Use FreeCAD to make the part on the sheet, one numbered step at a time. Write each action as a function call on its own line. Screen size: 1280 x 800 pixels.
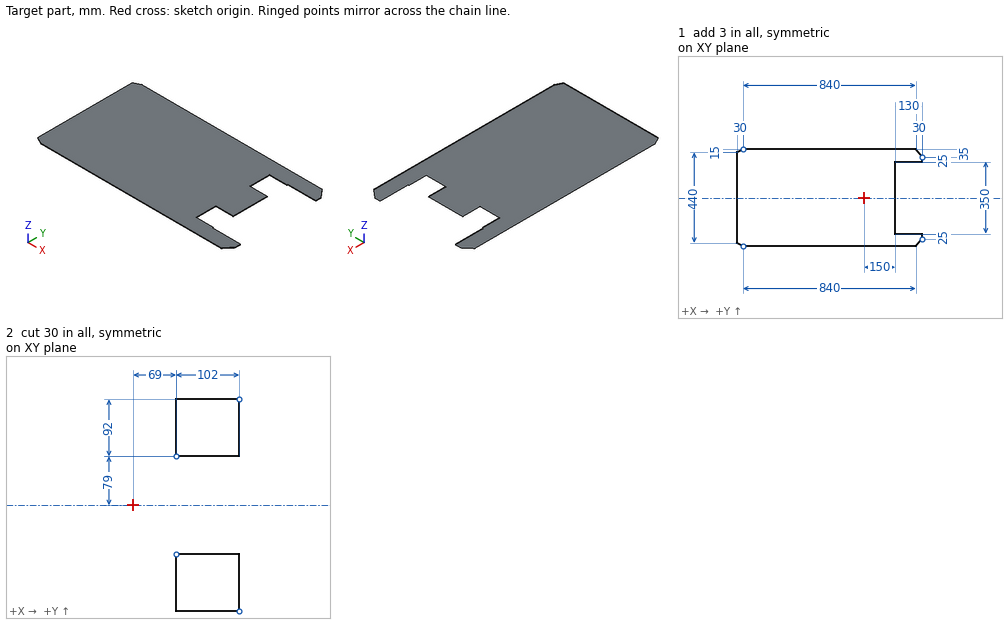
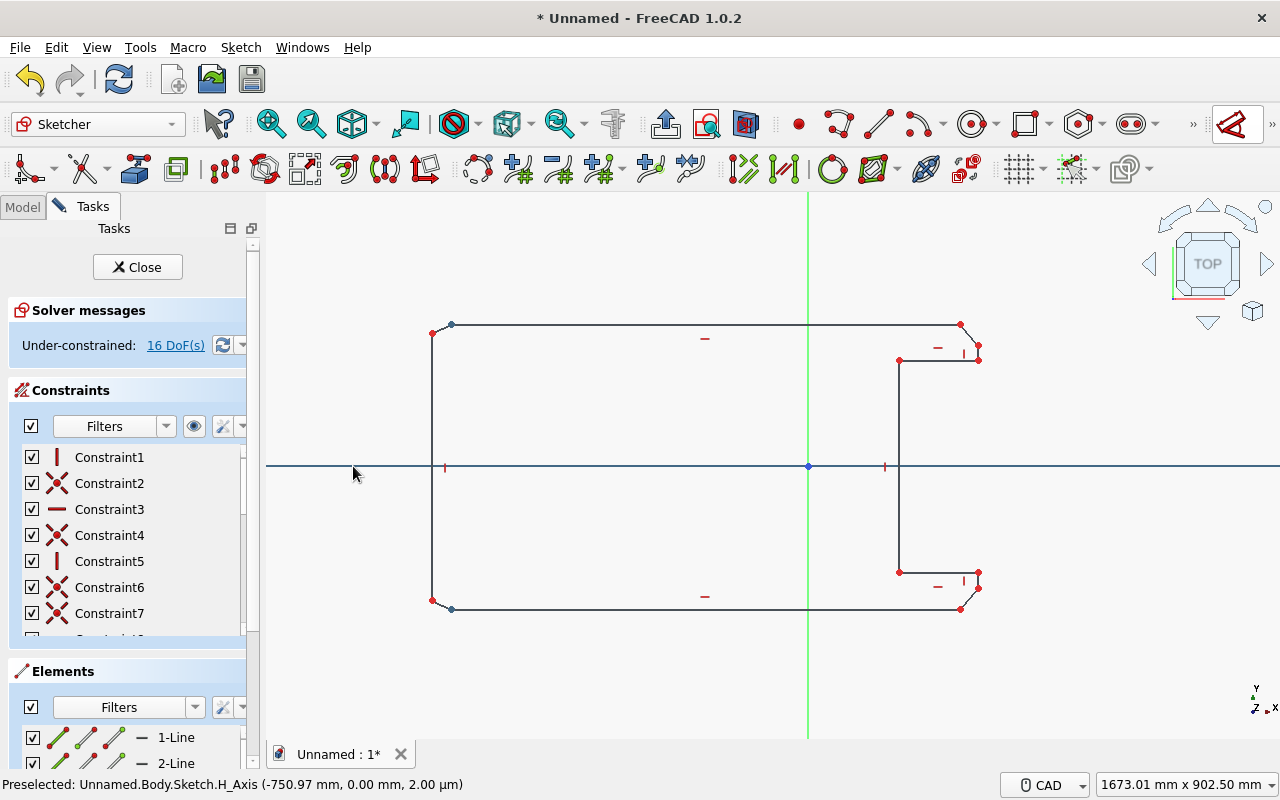
key(s)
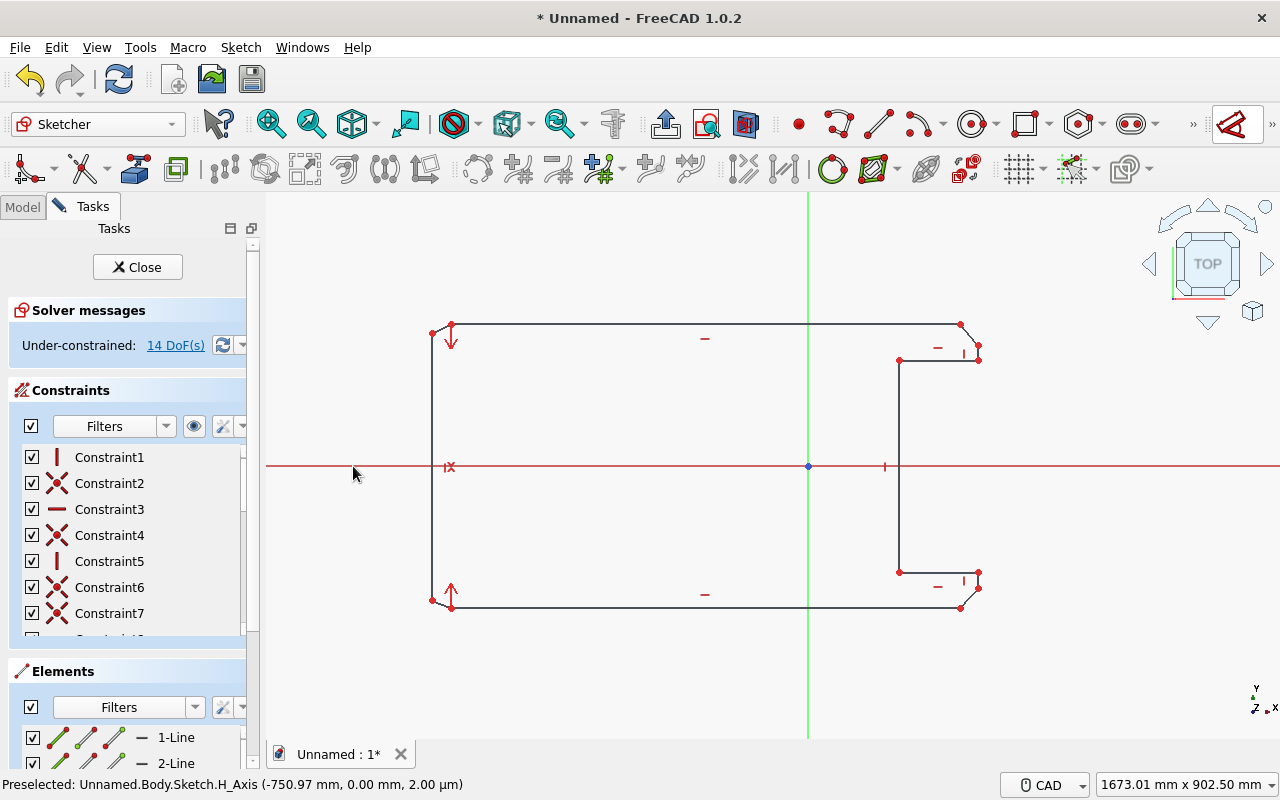
click(978, 346)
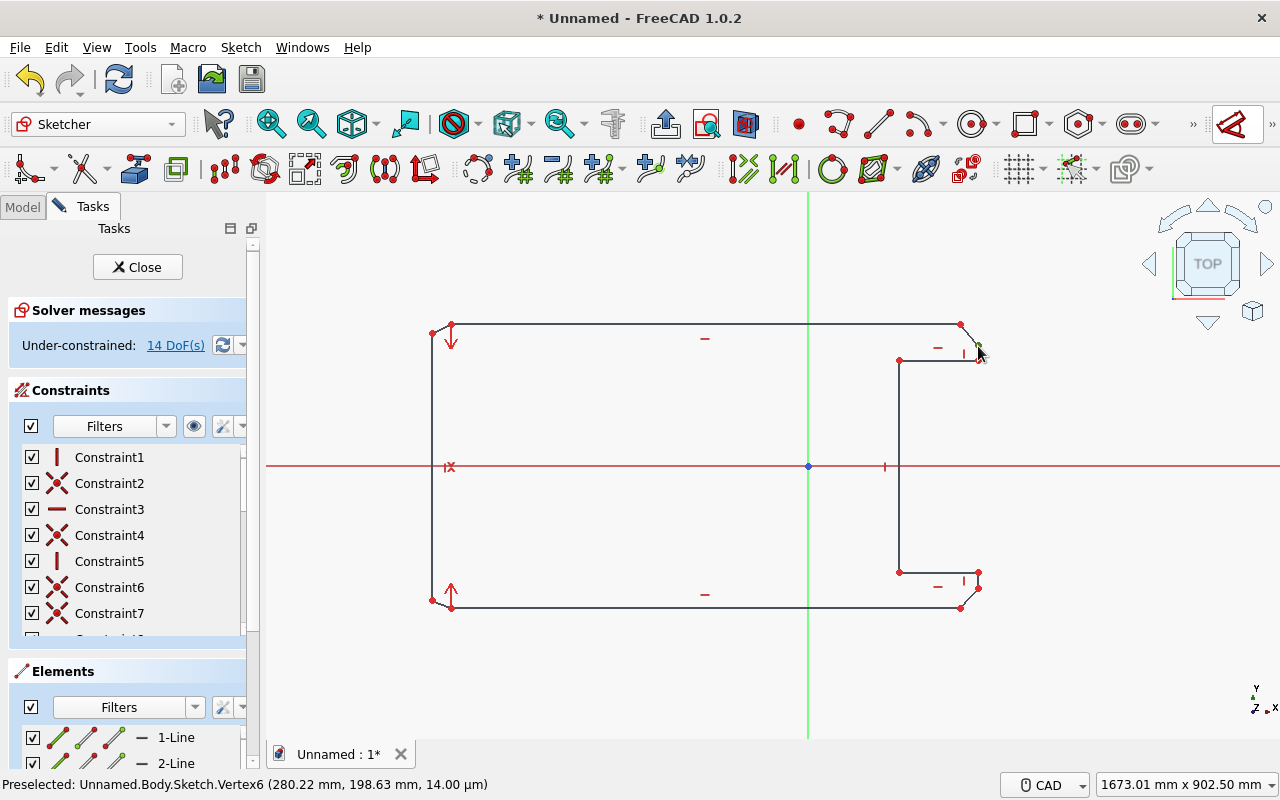
click(978, 589)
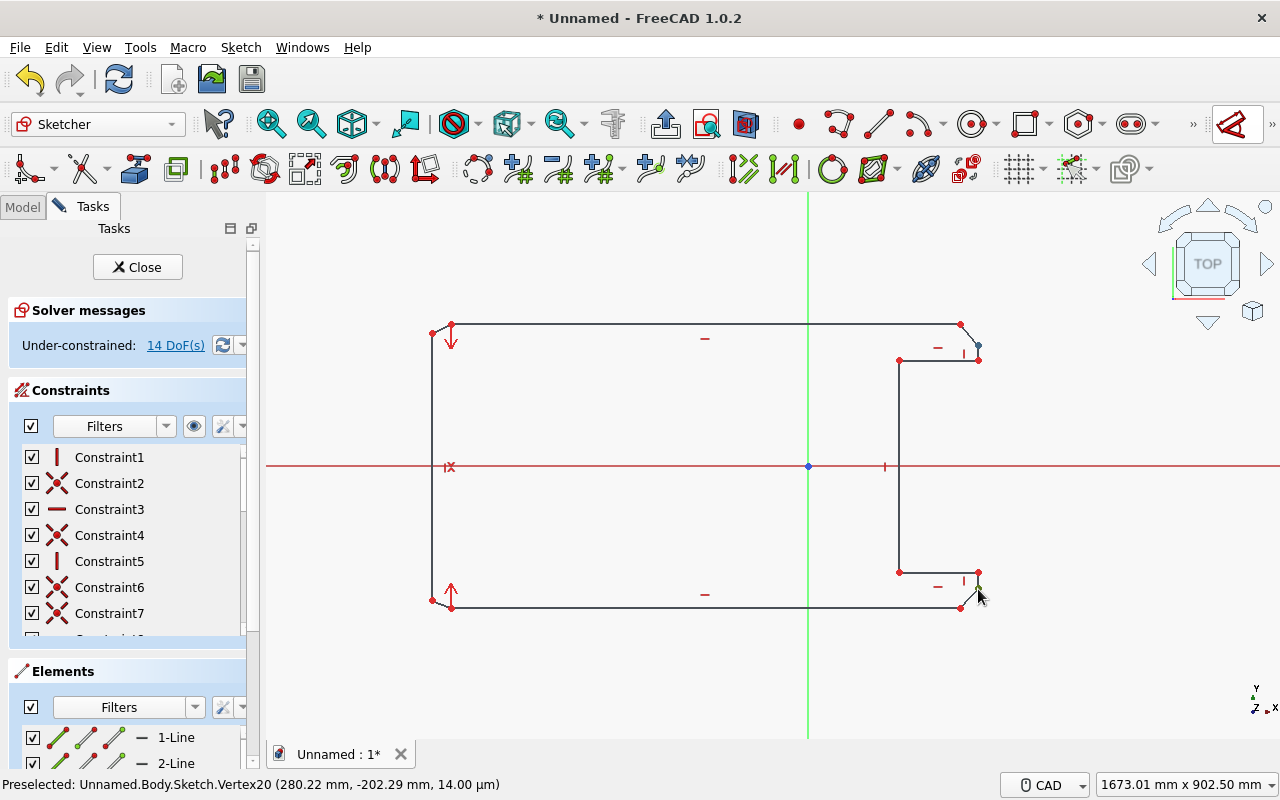
click(353, 466)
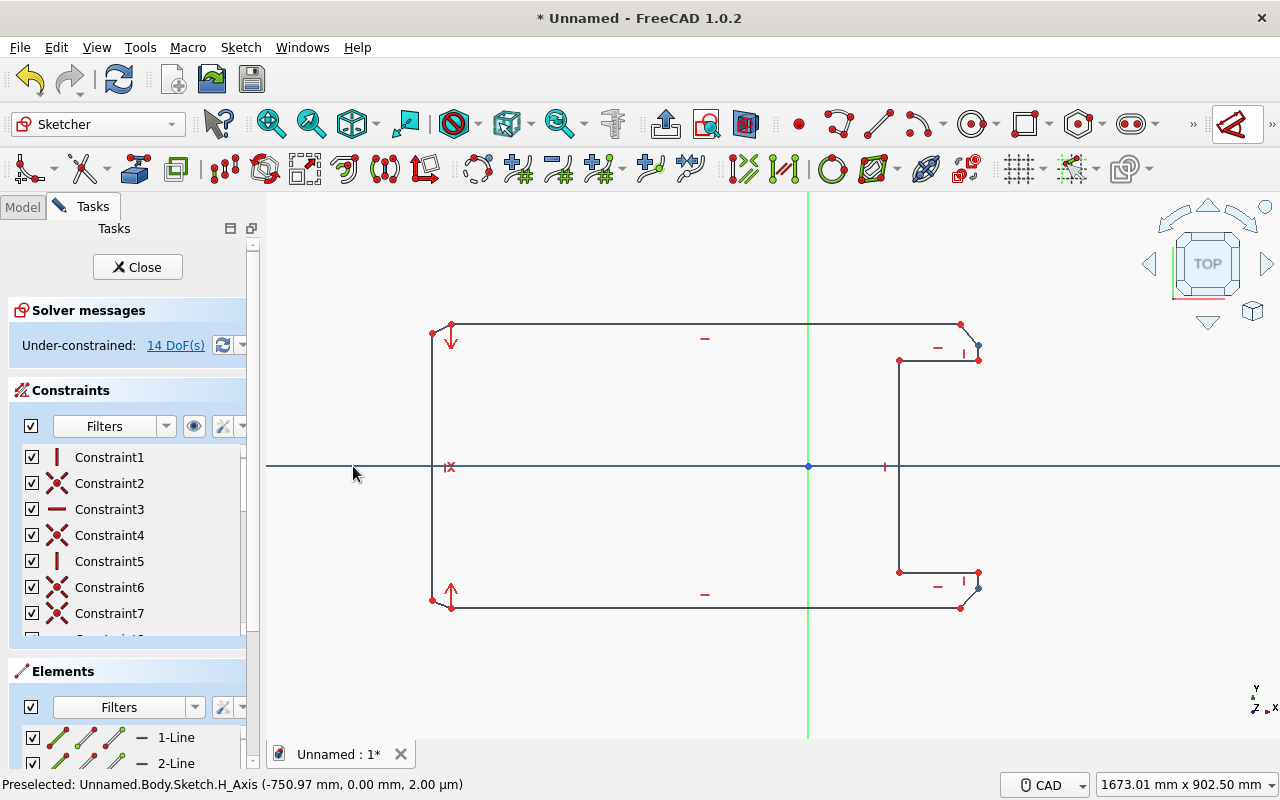
key(s)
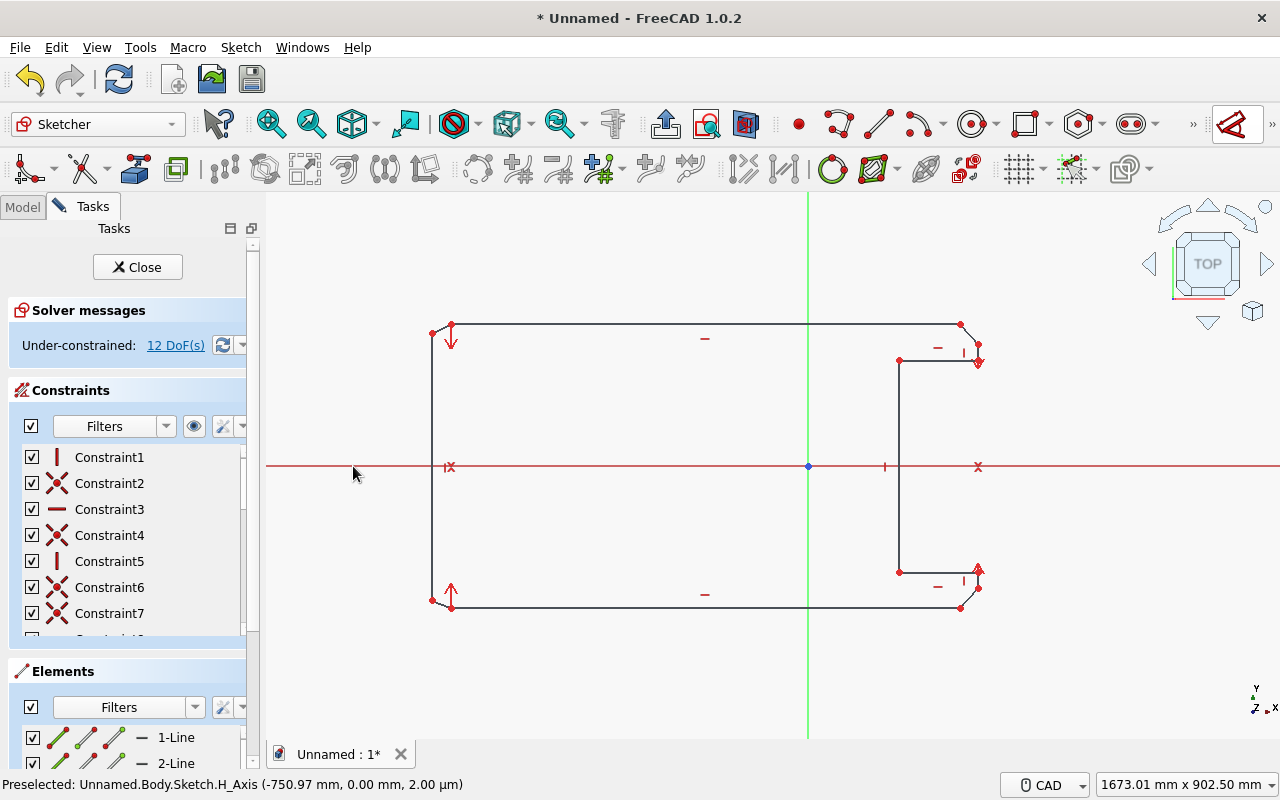
key(d)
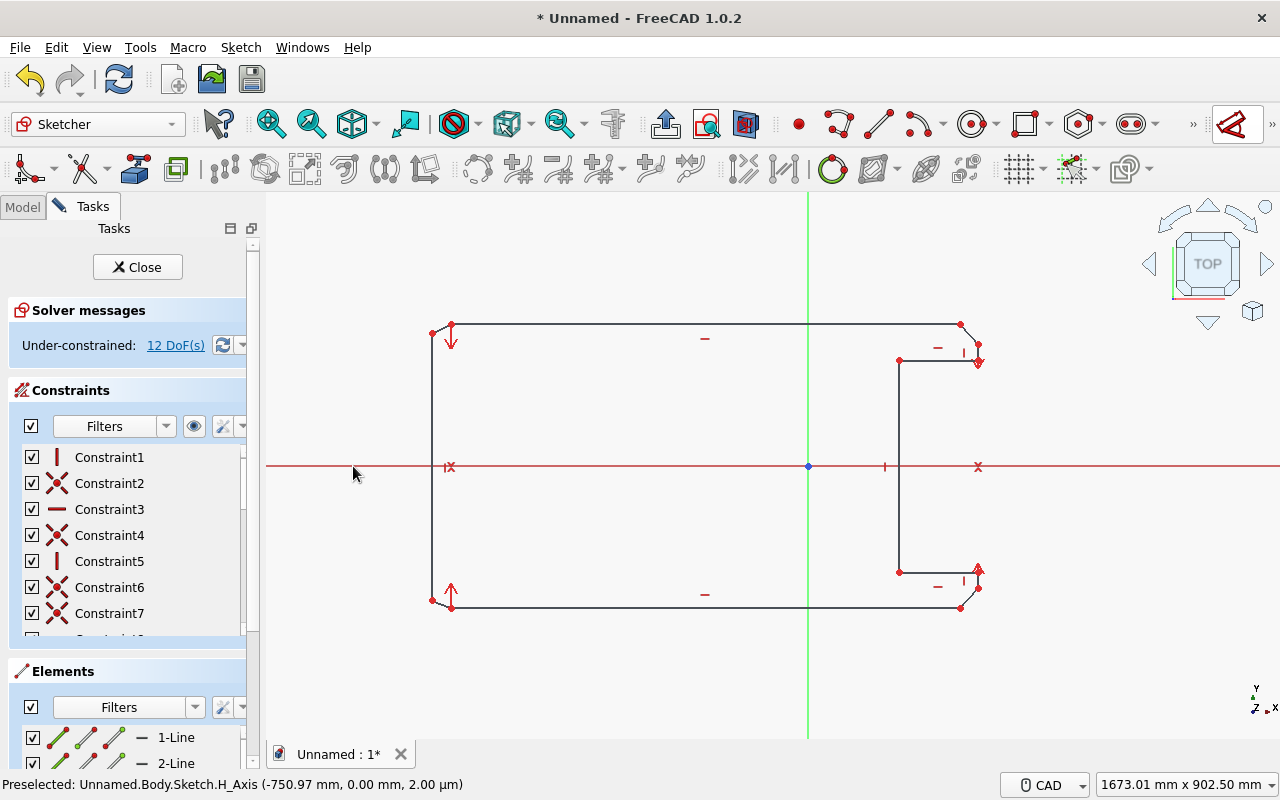
scroll(978, 353, up, 5)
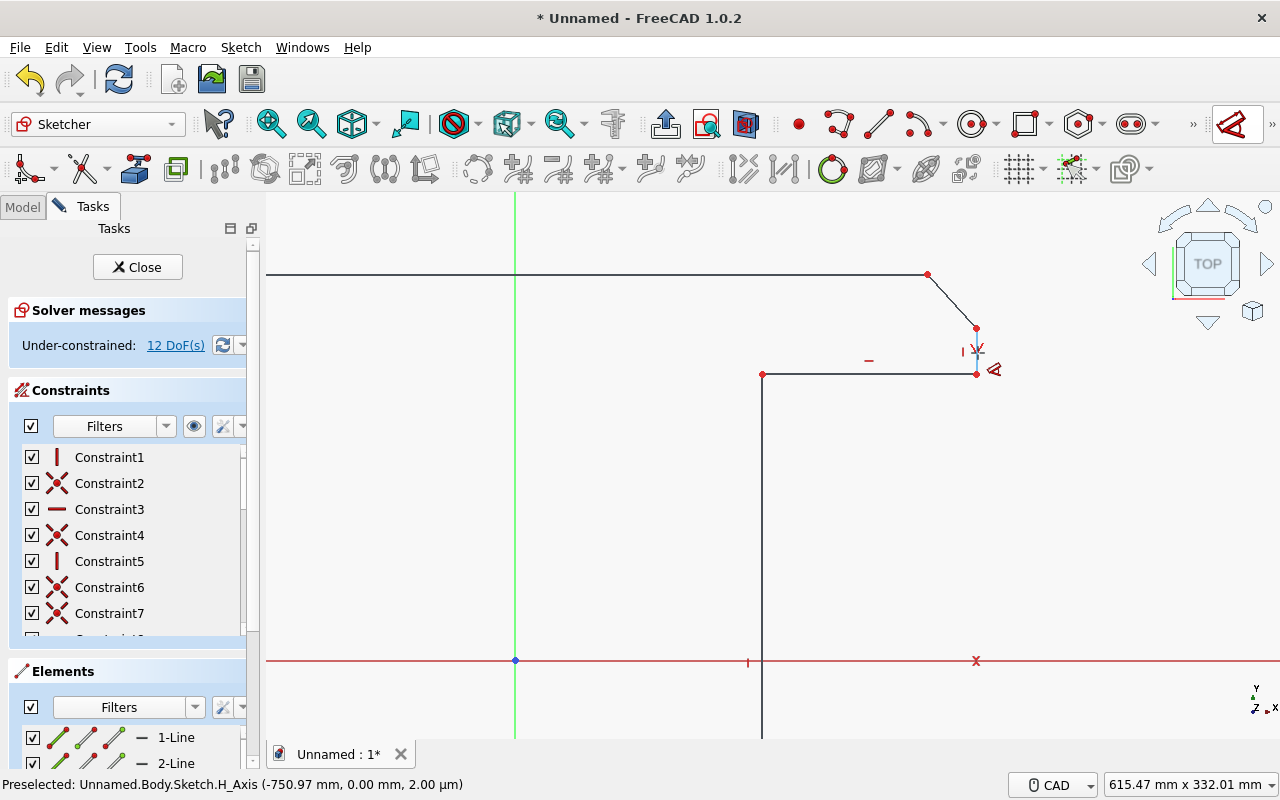
click(977, 352)
click(1011, 352)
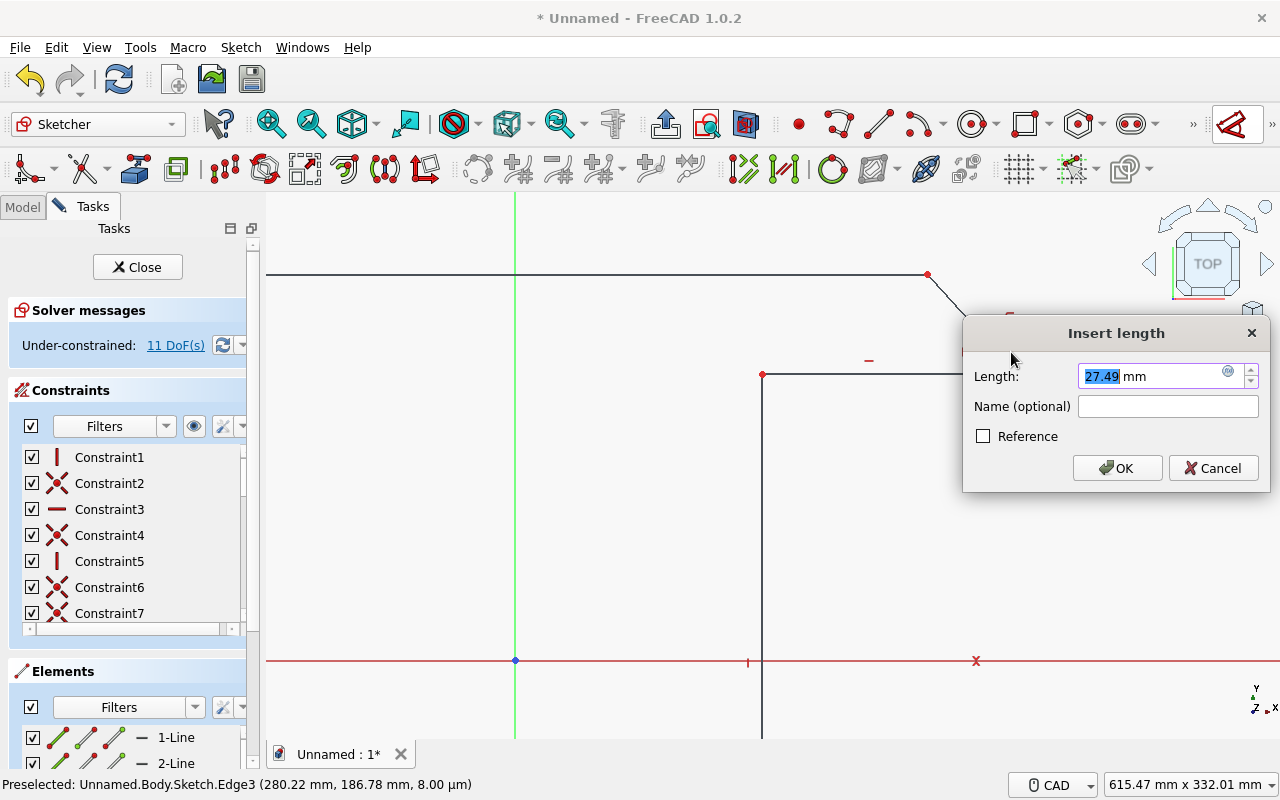
text(25)
key(Return)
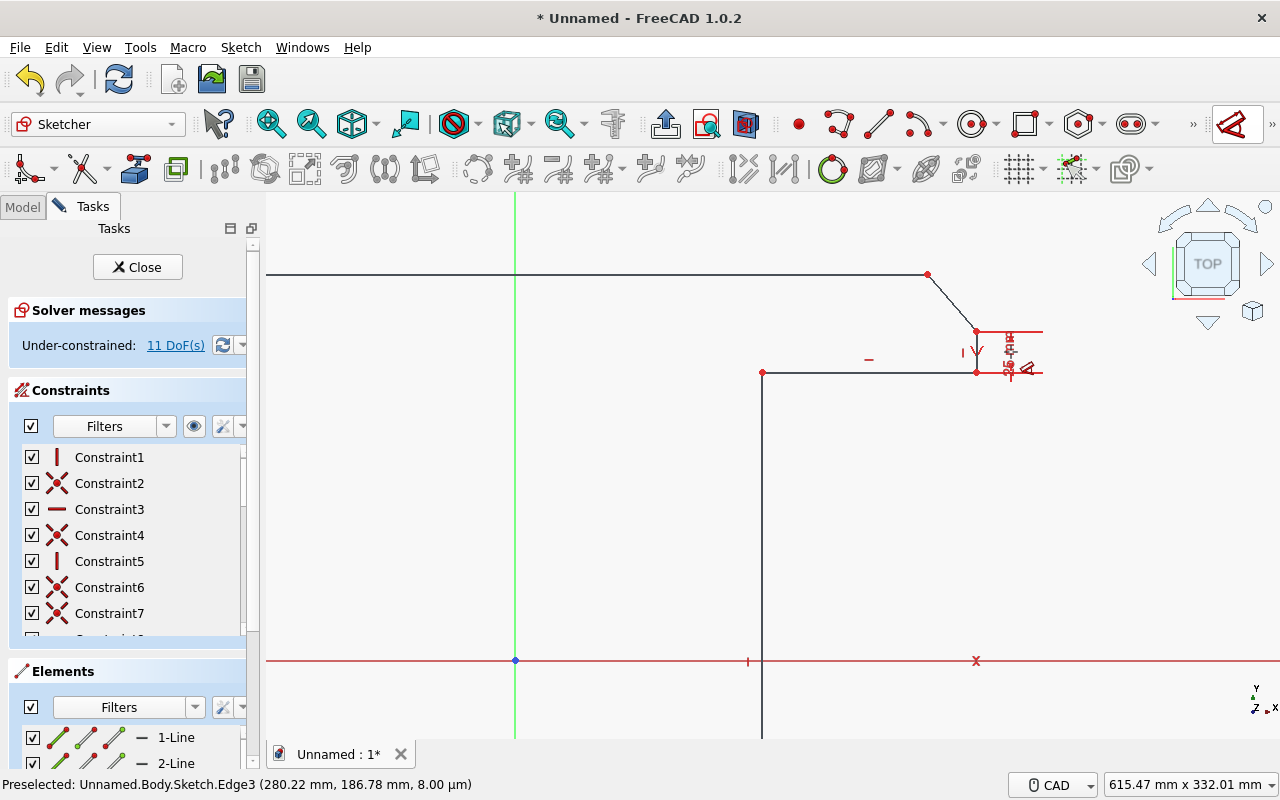
scroll(978, 352, down, 5)